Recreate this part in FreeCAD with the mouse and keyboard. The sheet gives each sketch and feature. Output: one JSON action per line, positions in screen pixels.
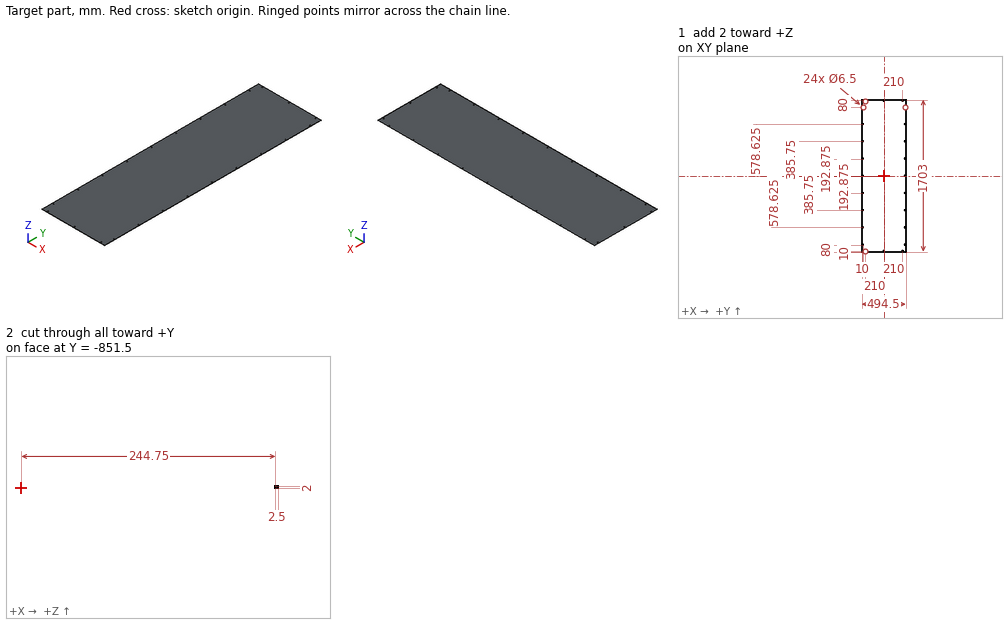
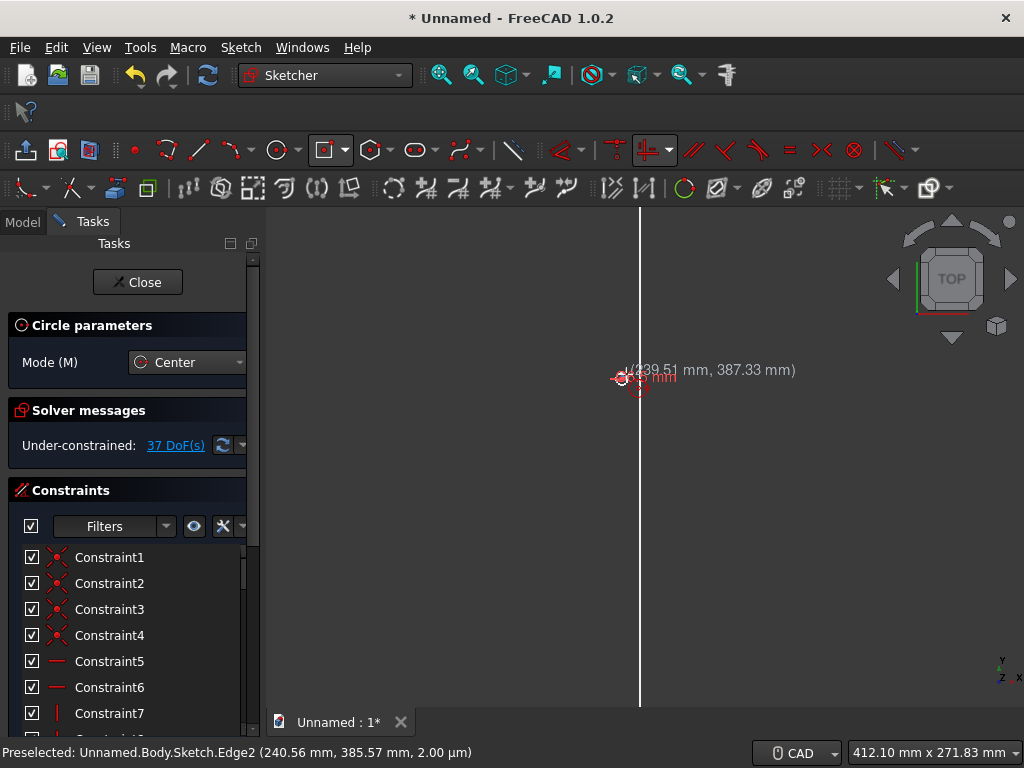
{"action": "scroll", "coordinate": [616, 394], "scroll_direction": "down", "scroll_amount": 12}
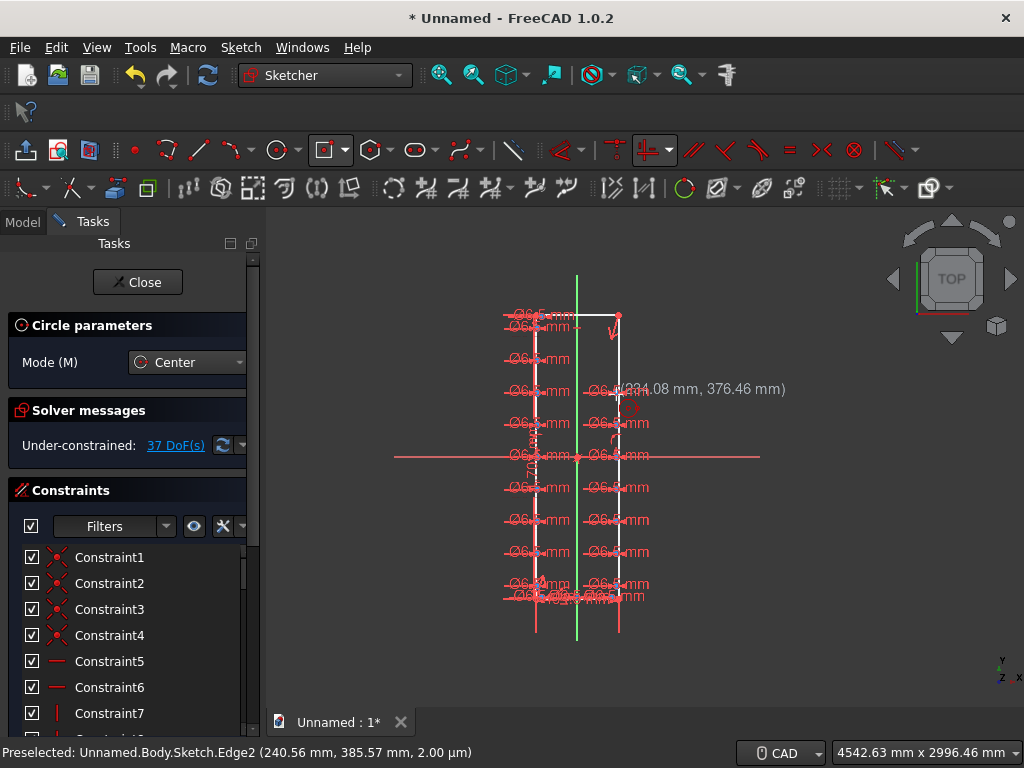
{"action": "scroll", "coordinate": [577, 317], "scroll_direction": "up", "scroll_amount": 19}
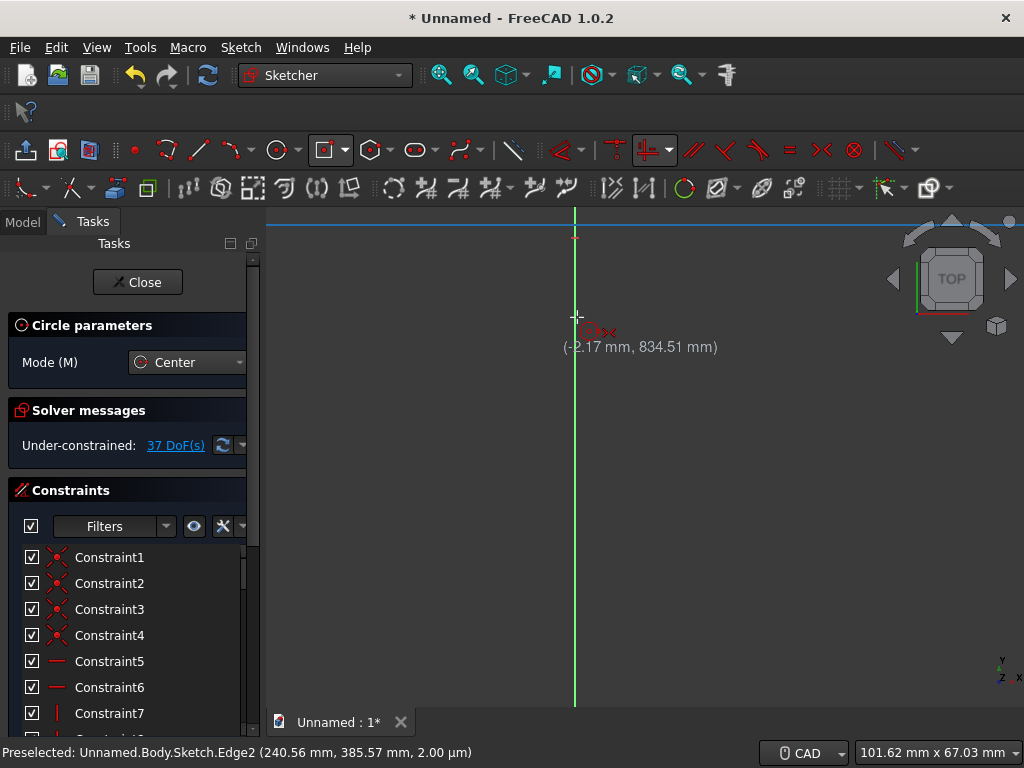
{"action": "scroll", "coordinate": [577, 285], "scroll_direction": "down", "scroll_amount": 18}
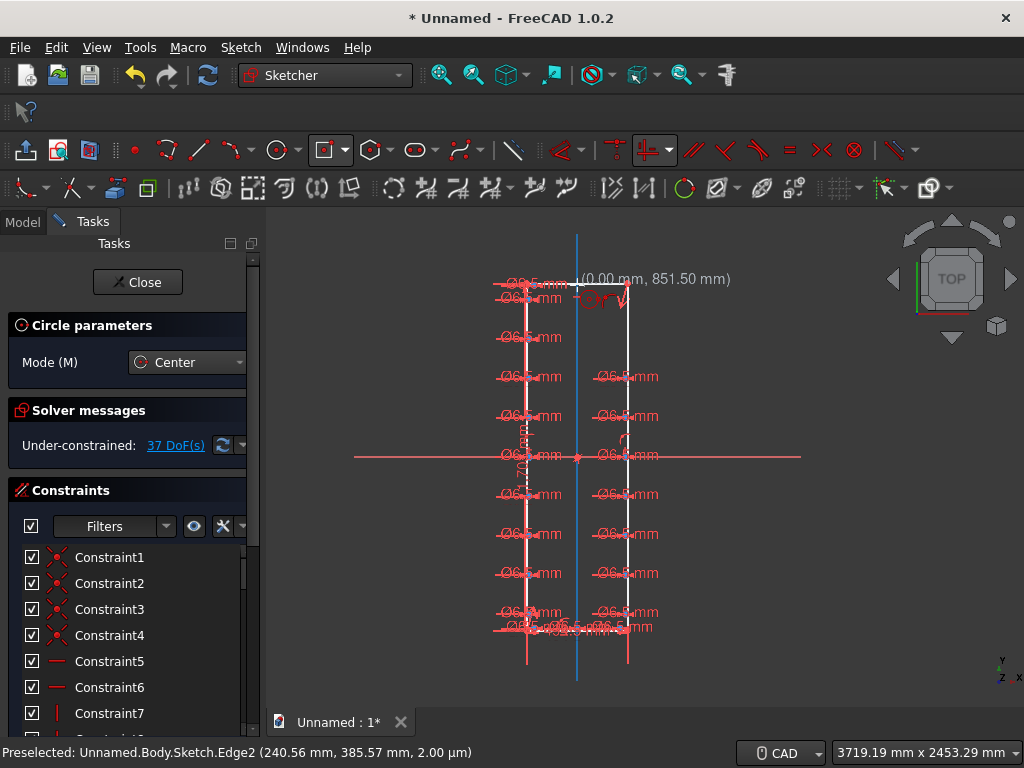
{"action": "scroll", "coordinate": [577, 286], "scroll_direction": "up", "scroll_amount": 11}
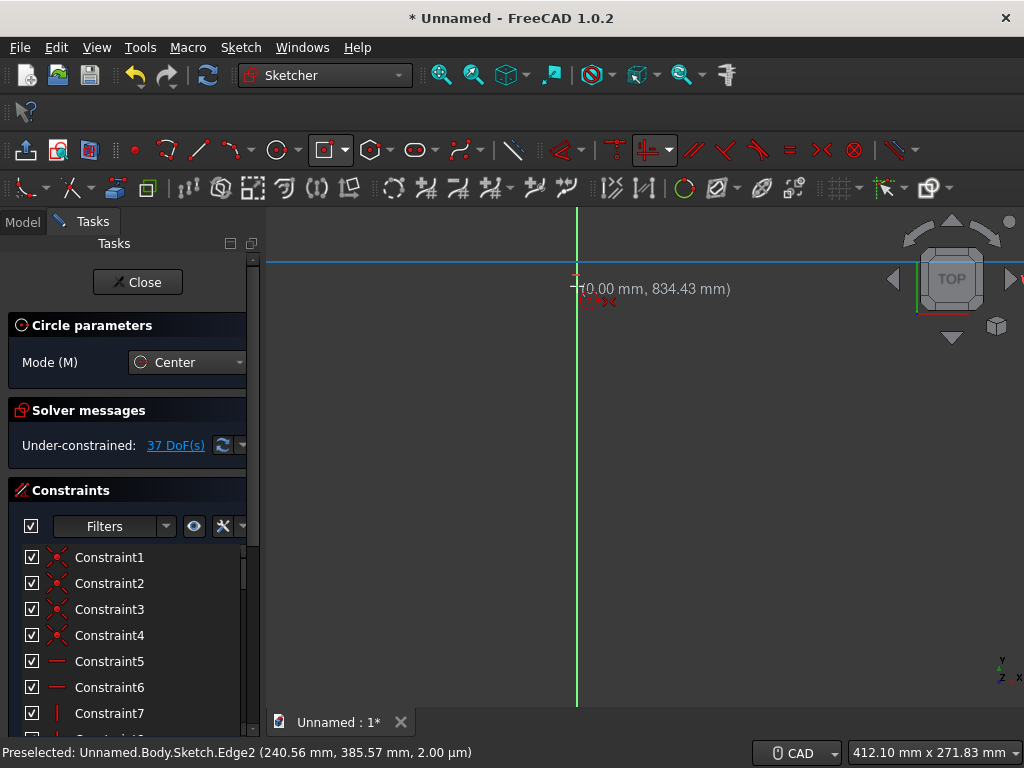
{"action": "left_click", "coordinate": [577, 281]}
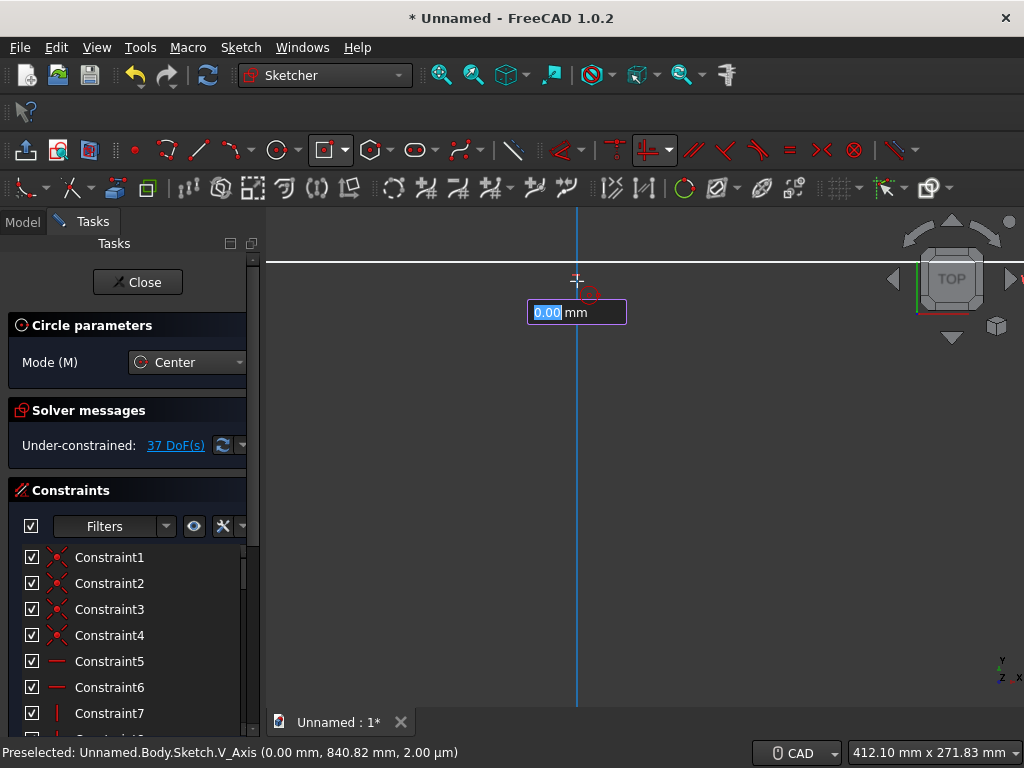
{"action": "scroll", "coordinate": [582, 279], "scroll_direction": "up", "scroll_amount": 6}
{"action": "mouse_move", "coordinate": [583, 278]}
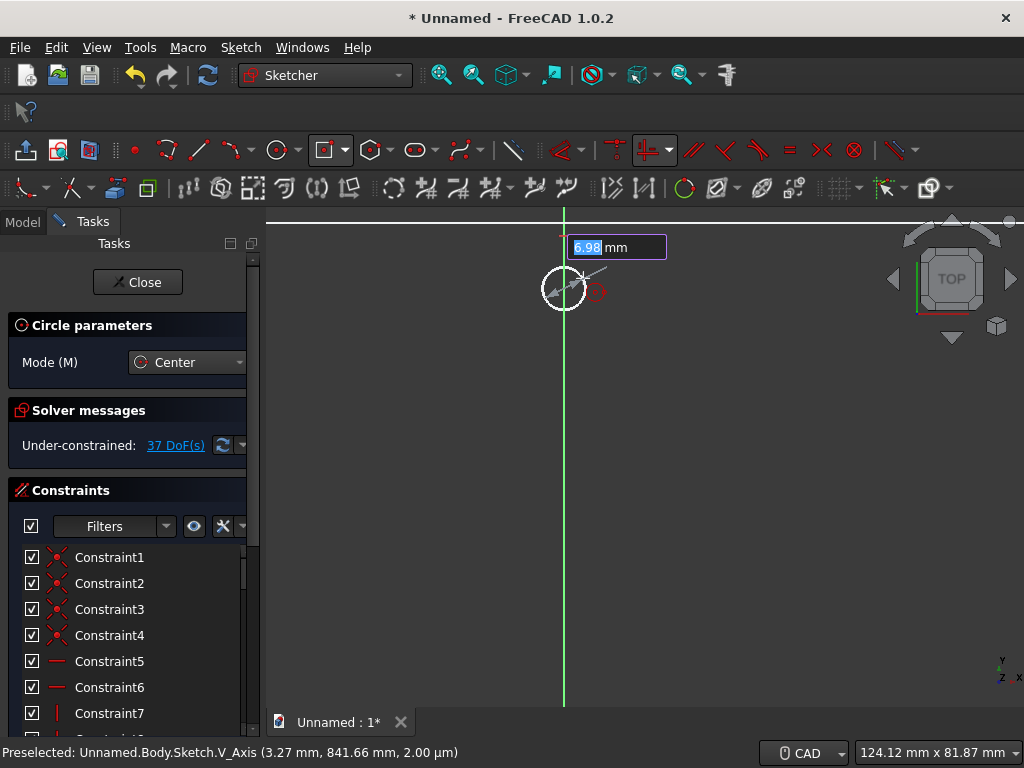
{"action": "type", "text": "6.5"}
{"action": "key", "text": "Return"}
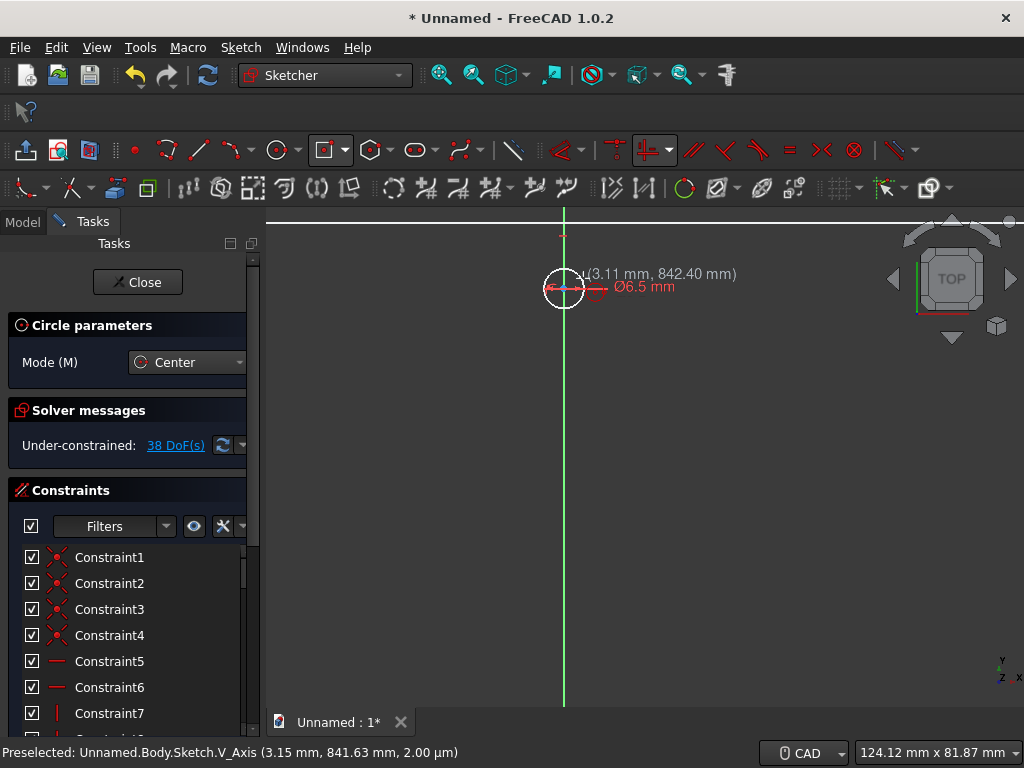
{"action": "scroll", "coordinate": [577, 286], "scroll_direction": "down", "scroll_amount": 17}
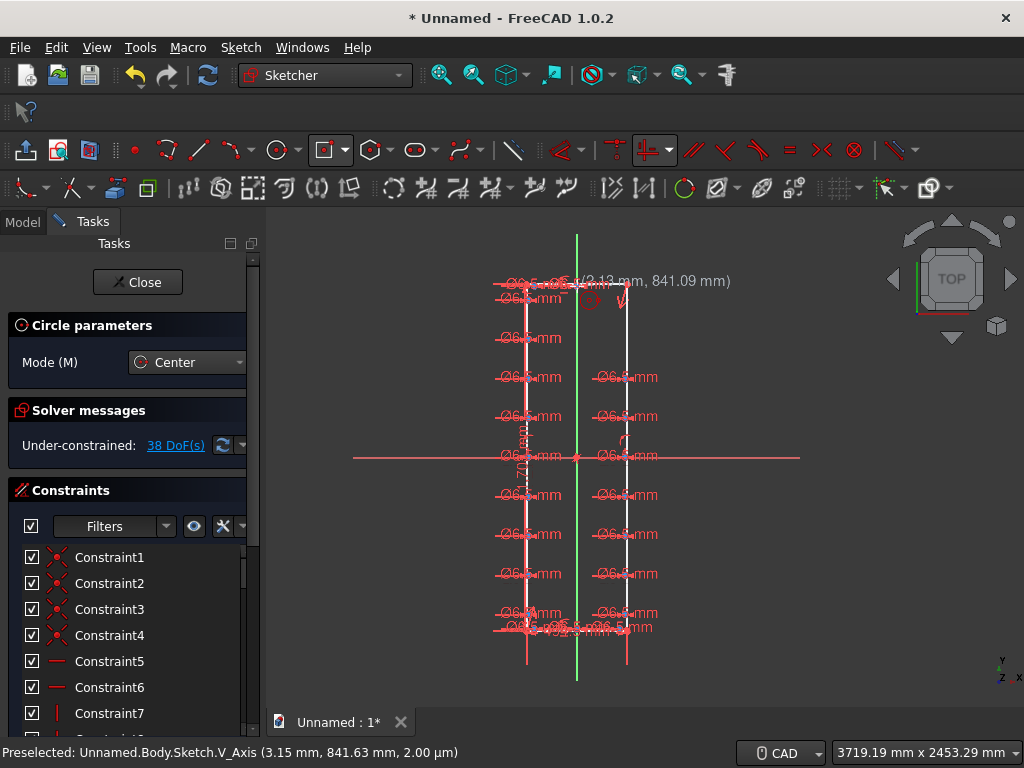
{"action": "scroll", "coordinate": [625, 340], "scroll_direction": "up", "scroll_amount": 18}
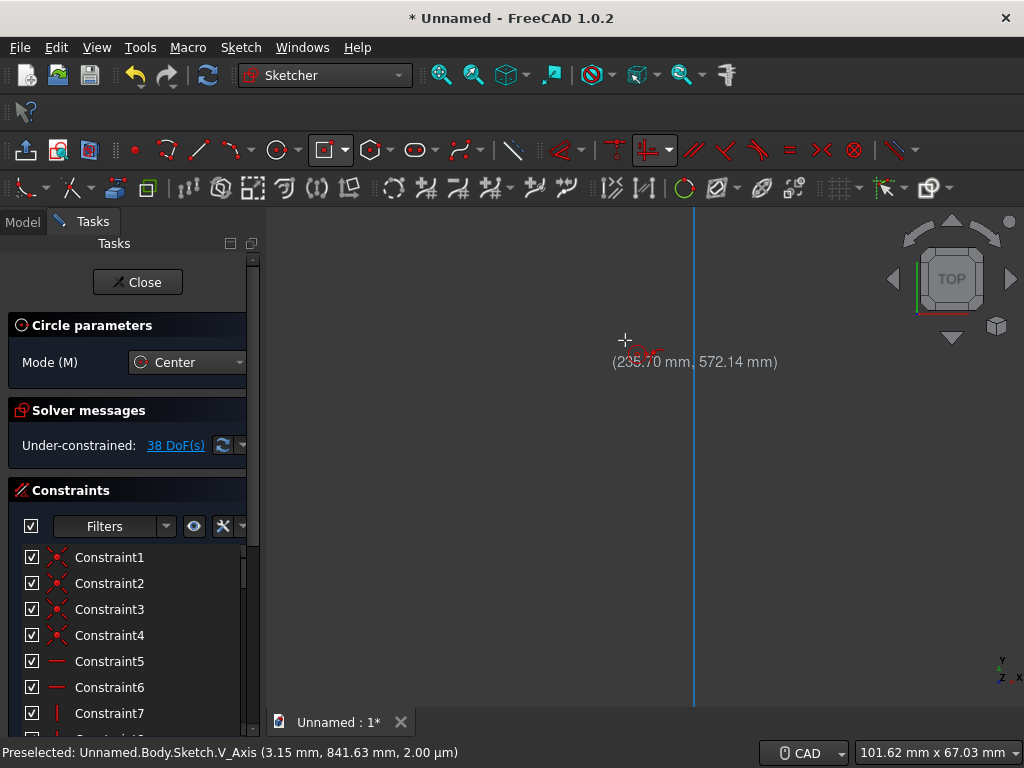
{"action": "scroll", "coordinate": [625, 340], "scroll_direction": "down", "scroll_amount": 18}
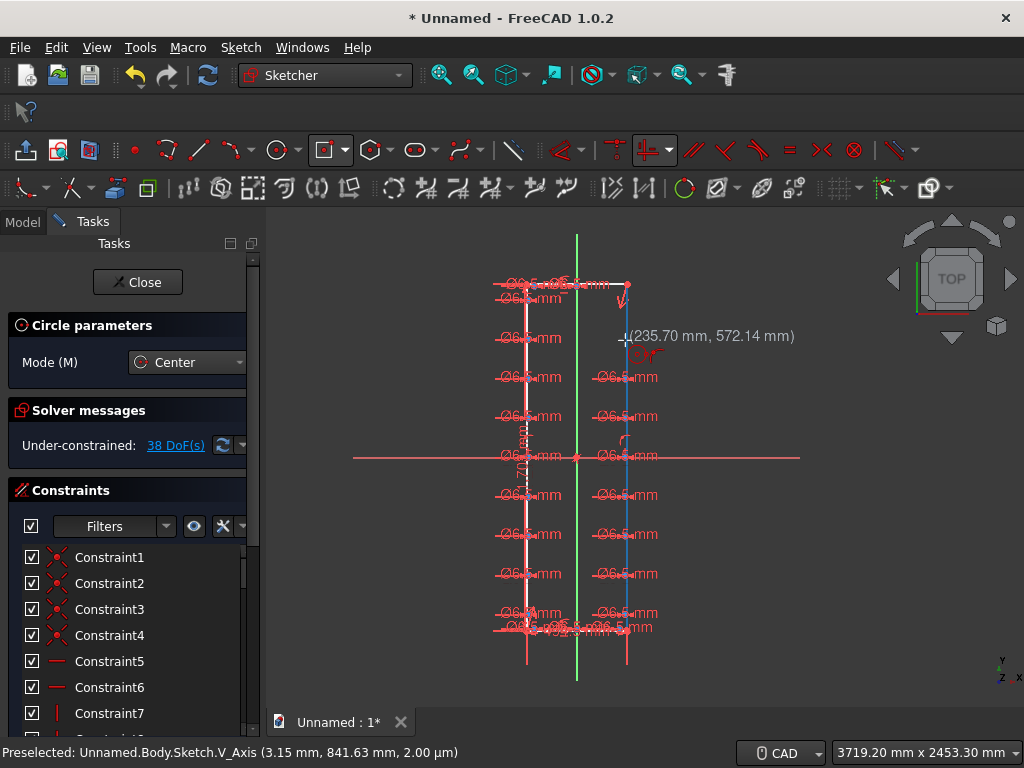
{"action": "scroll", "coordinate": [625, 340], "scroll_direction": "up", "scroll_amount": 11}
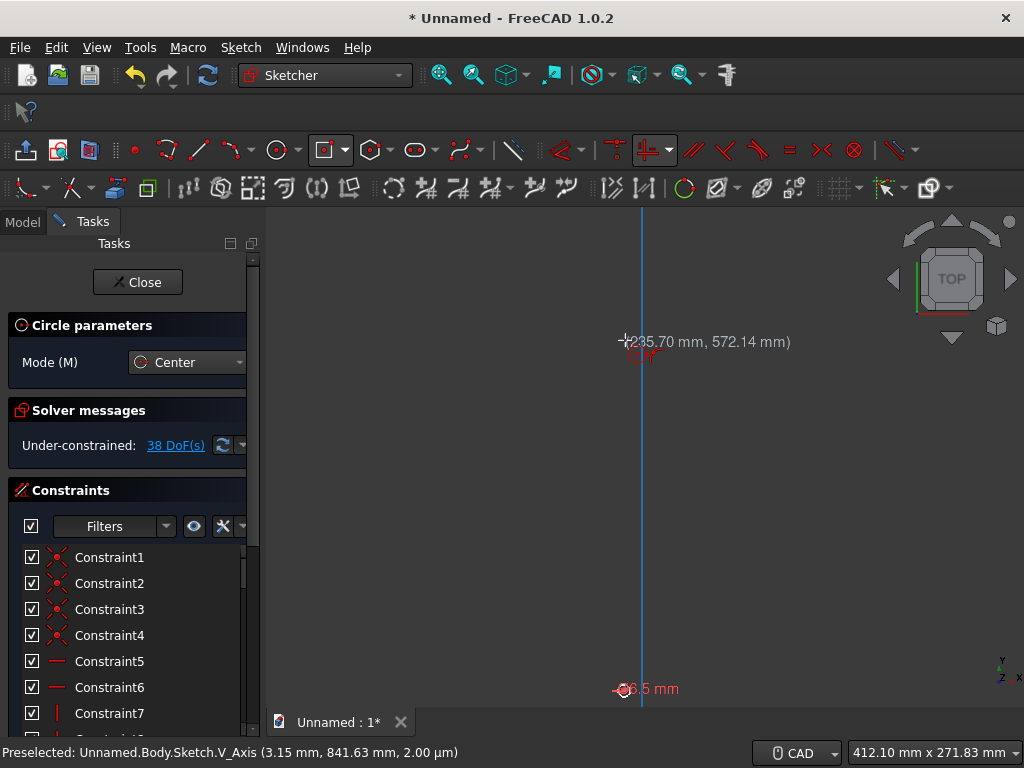
{"action": "left_click", "coordinate": [624, 335]}
{"action": "mouse_move", "coordinate": [628, 331]}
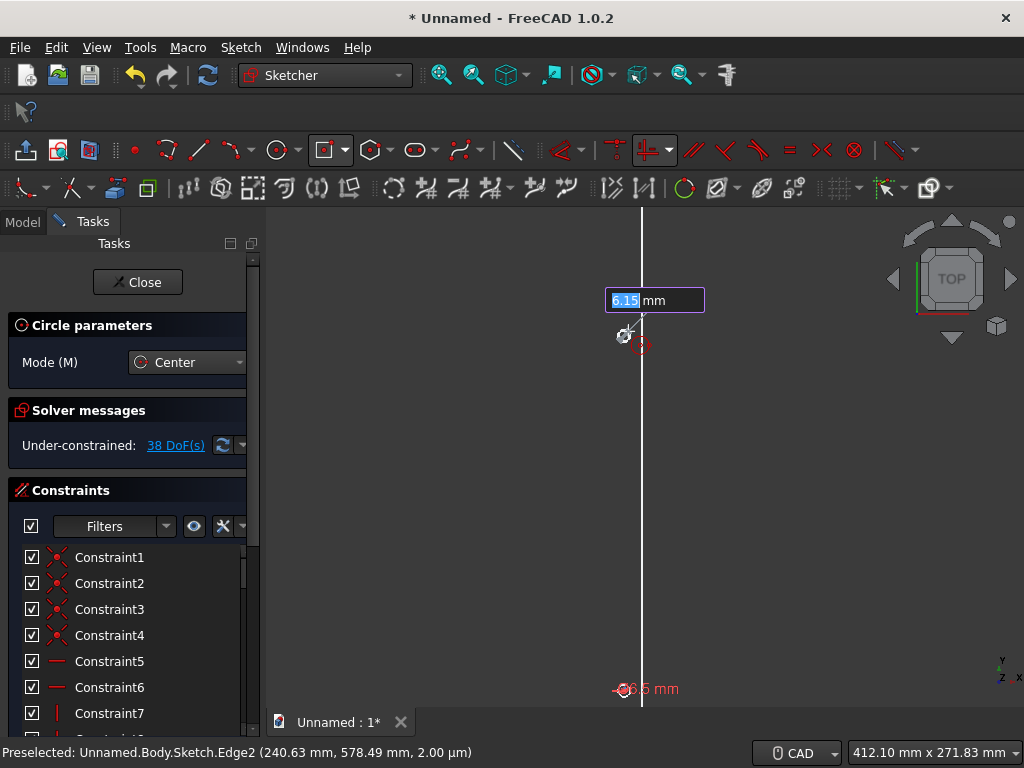
{"action": "type", "text": "6.5"}
{"action": "key", "text": "Return"}